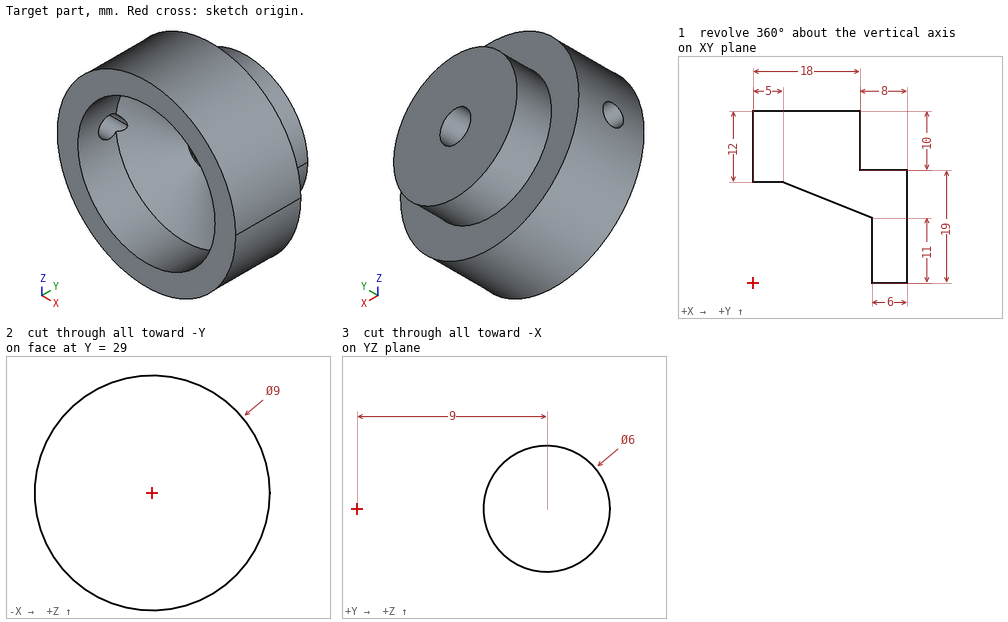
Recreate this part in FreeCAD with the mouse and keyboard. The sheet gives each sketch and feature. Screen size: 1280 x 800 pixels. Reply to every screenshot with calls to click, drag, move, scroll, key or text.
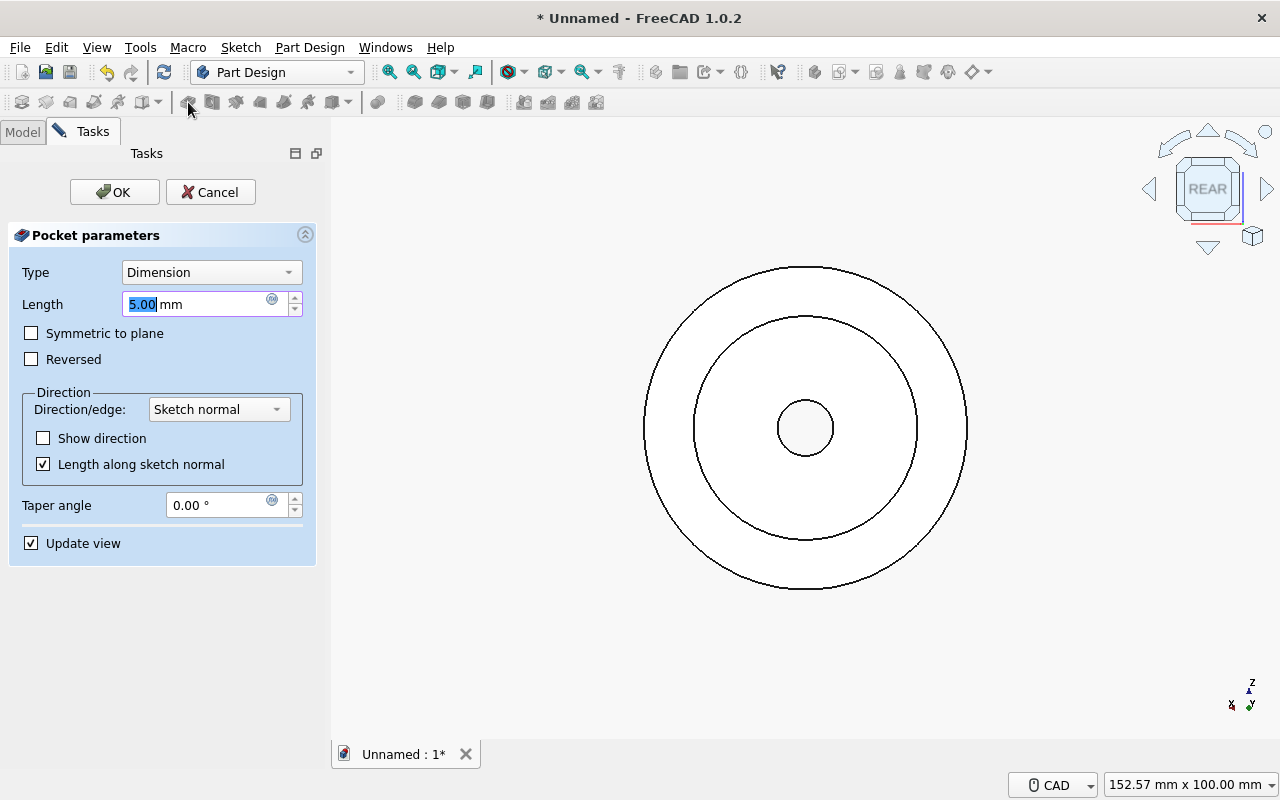
click(212, 272)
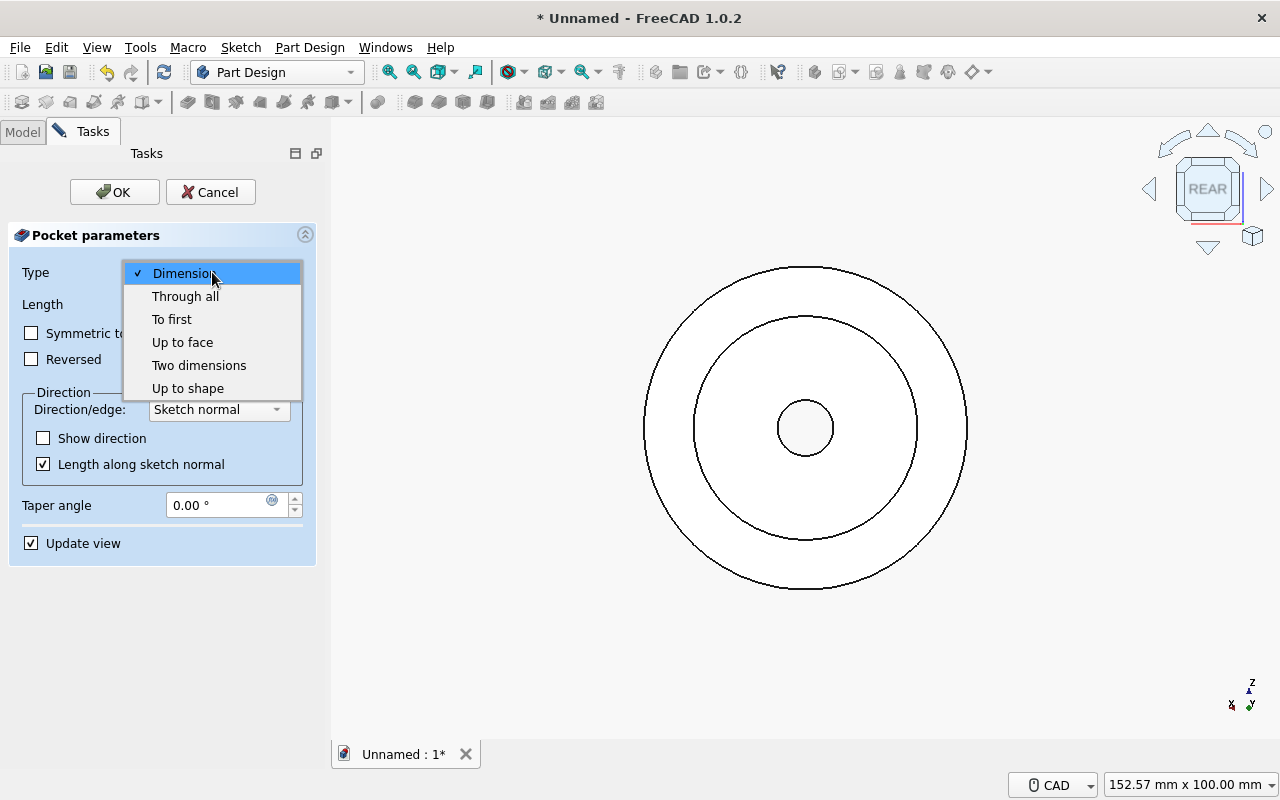
click(212, 296)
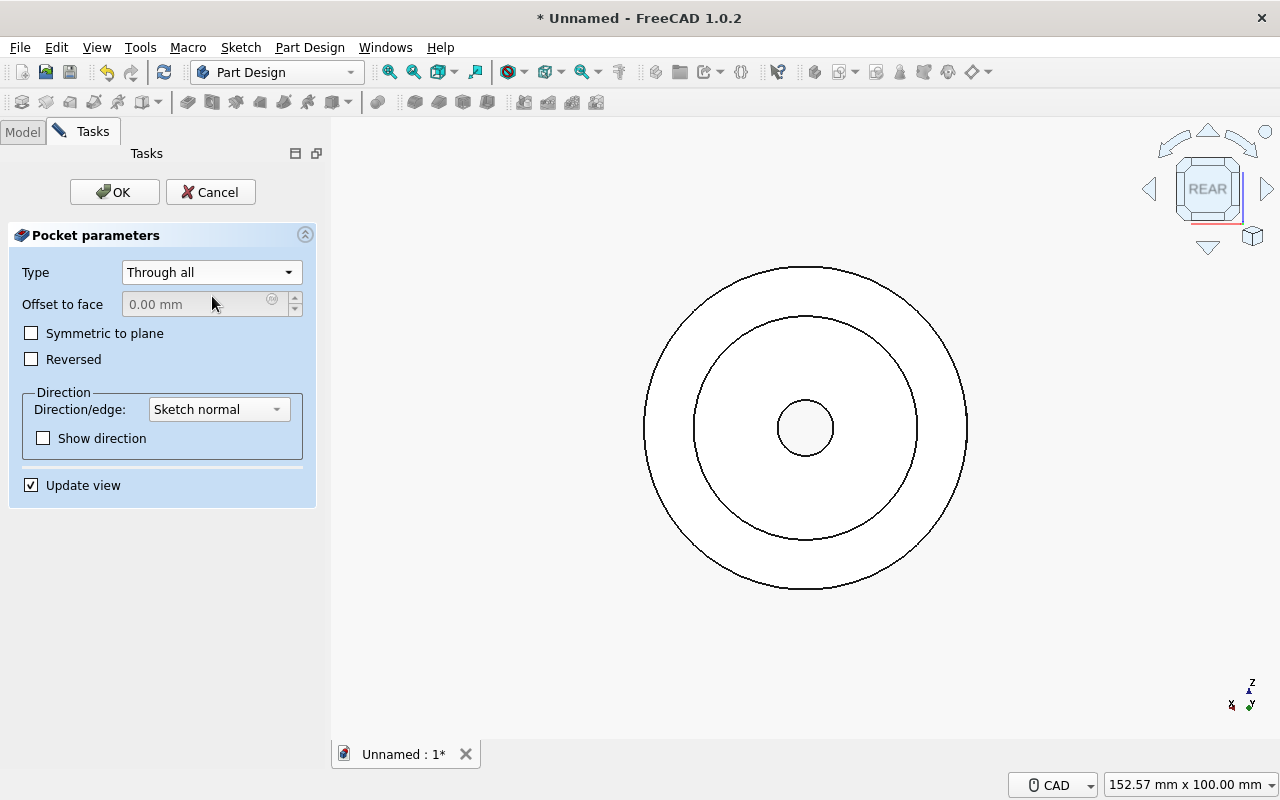
click(115, 192)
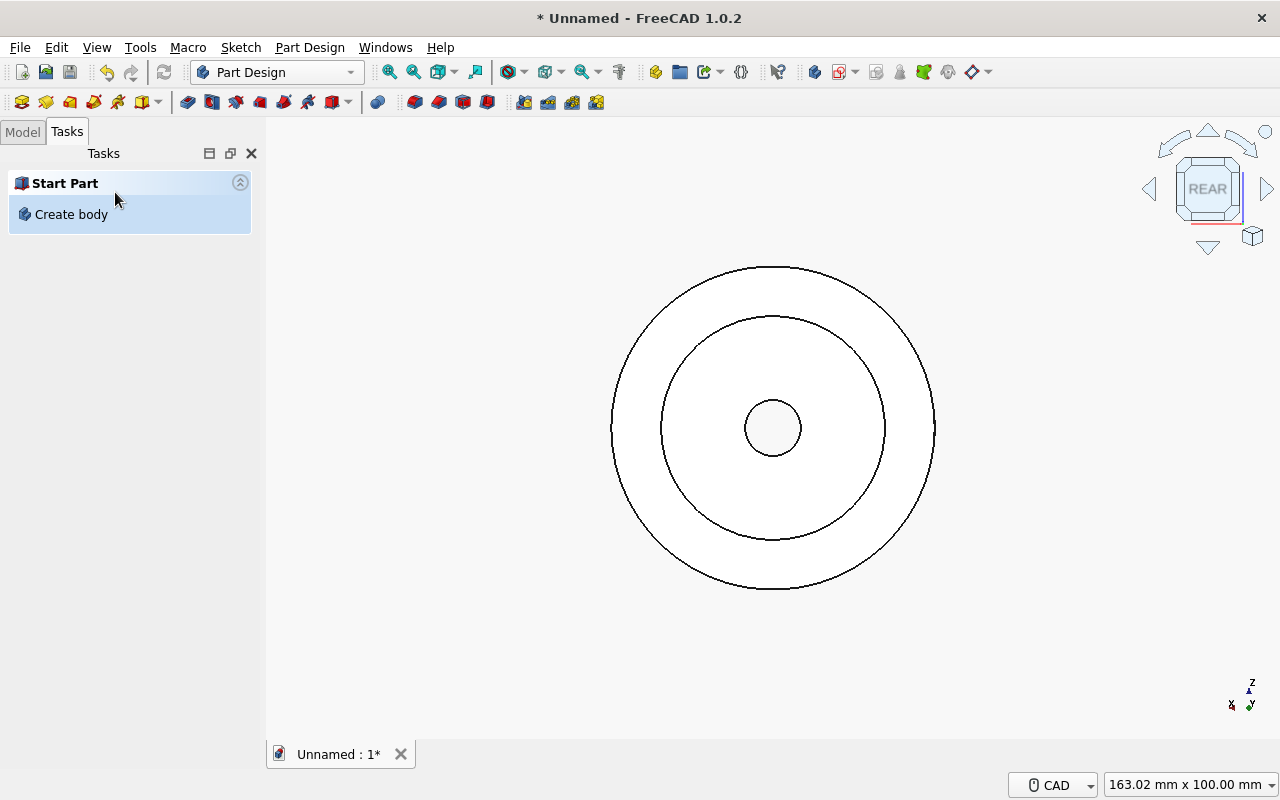
key(0)